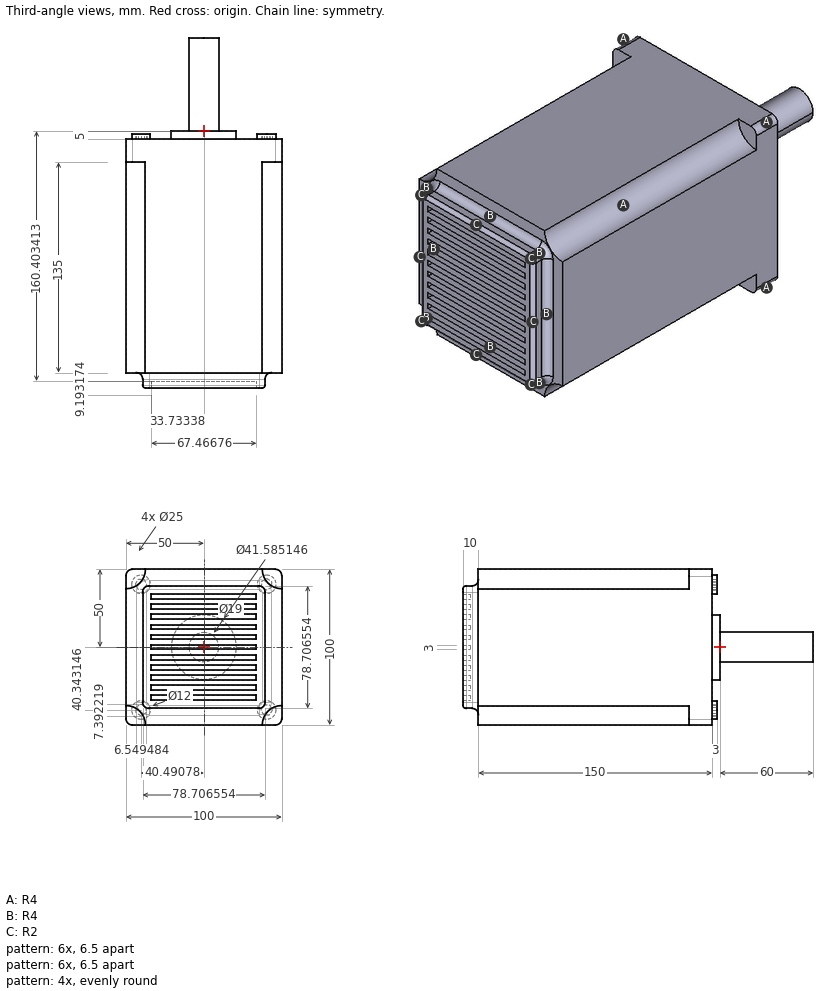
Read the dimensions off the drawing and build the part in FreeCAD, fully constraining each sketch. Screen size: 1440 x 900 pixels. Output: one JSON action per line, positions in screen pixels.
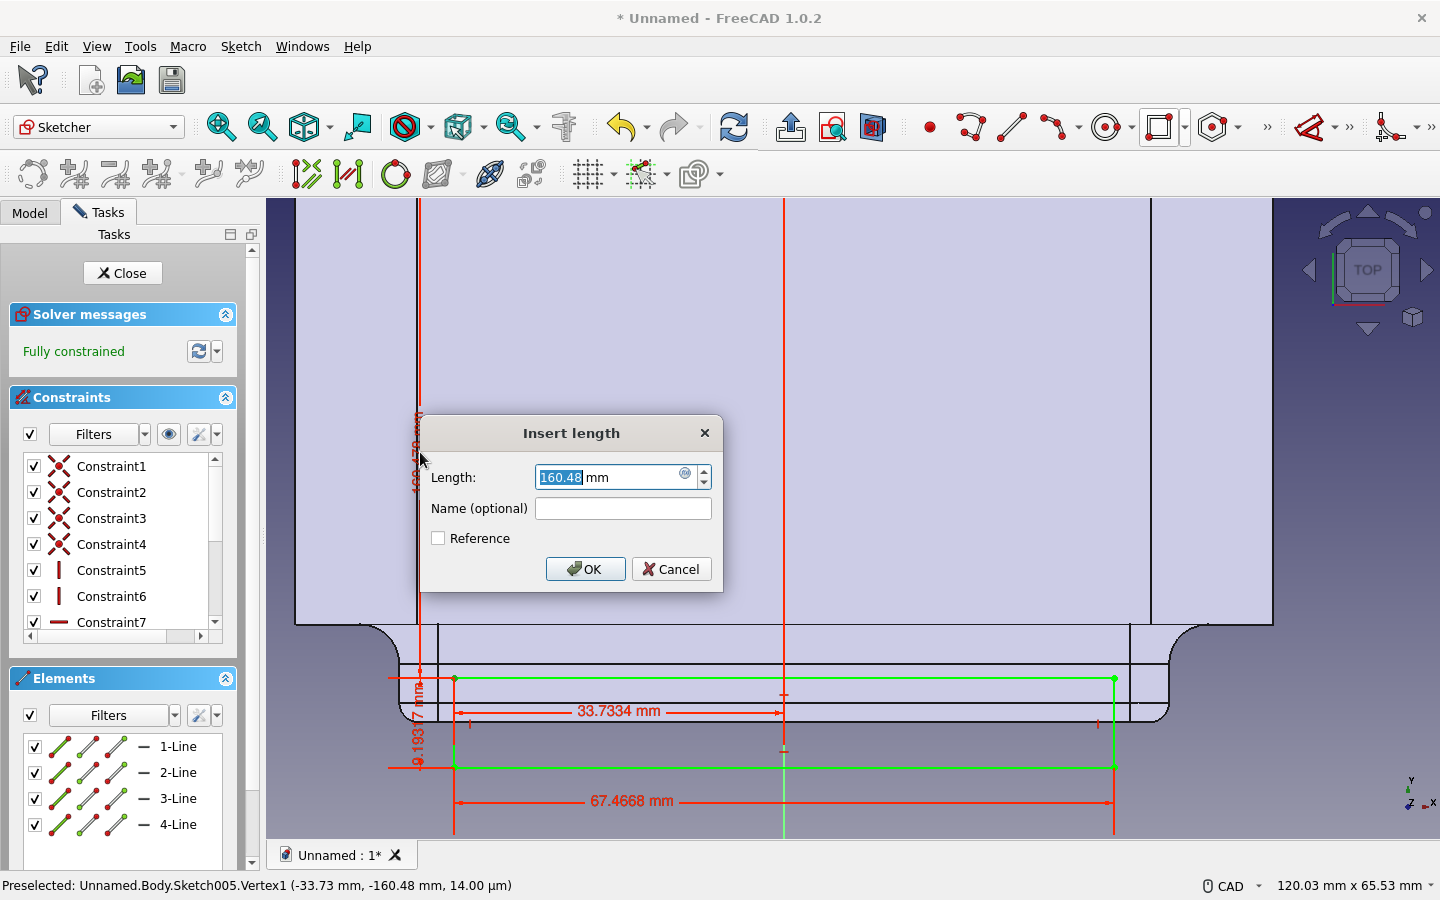
{"action": "type", "text": "160.403413"}
{"action": "key", "text": "Return"}
{"action": "key", "text": "Escape"}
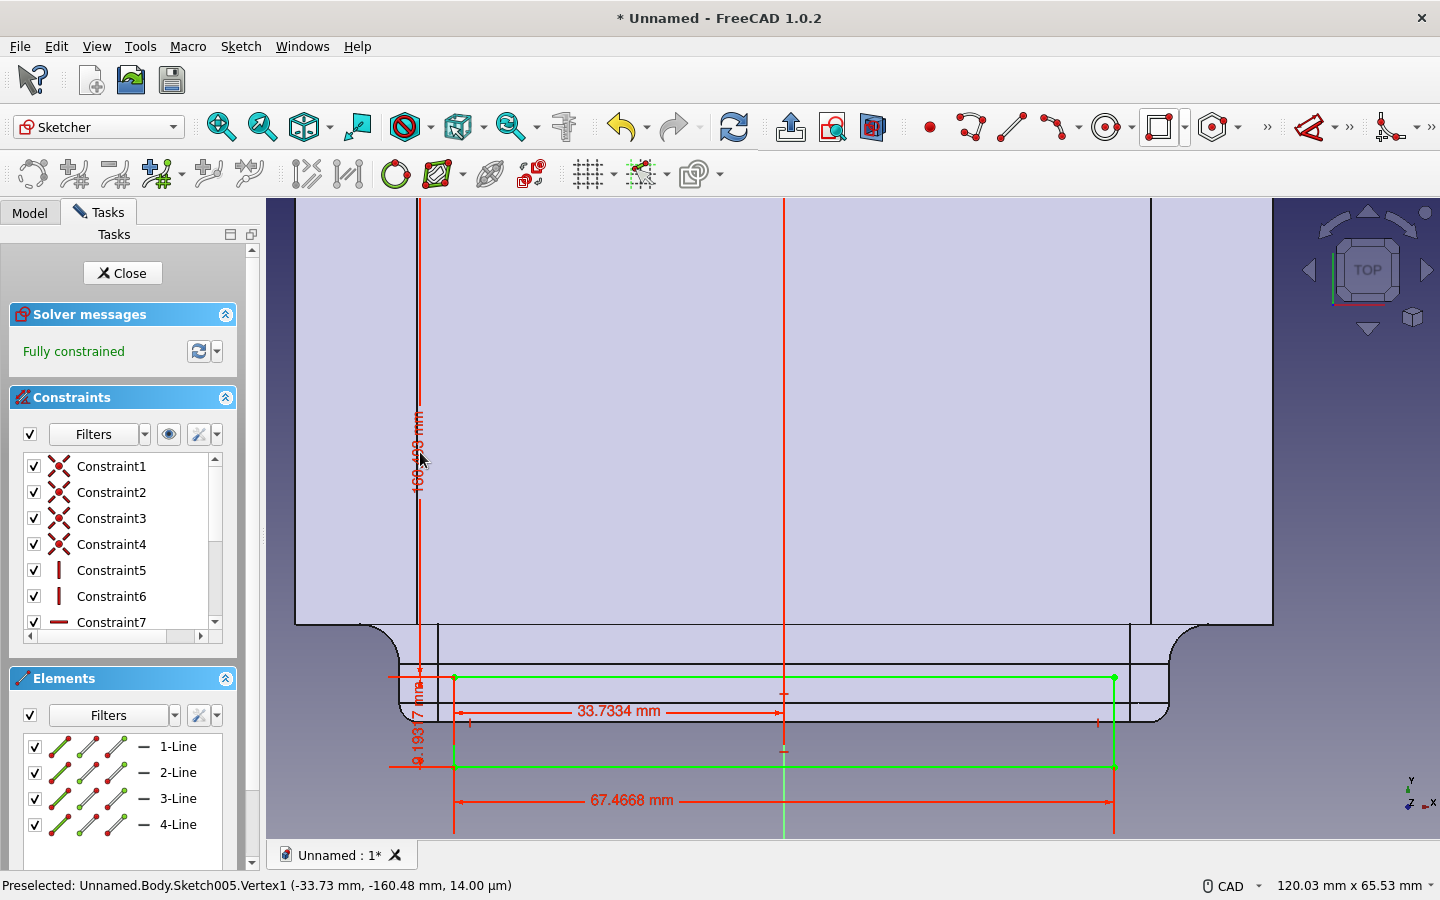
{"action": "left_click", "coordinate": [123, 273]}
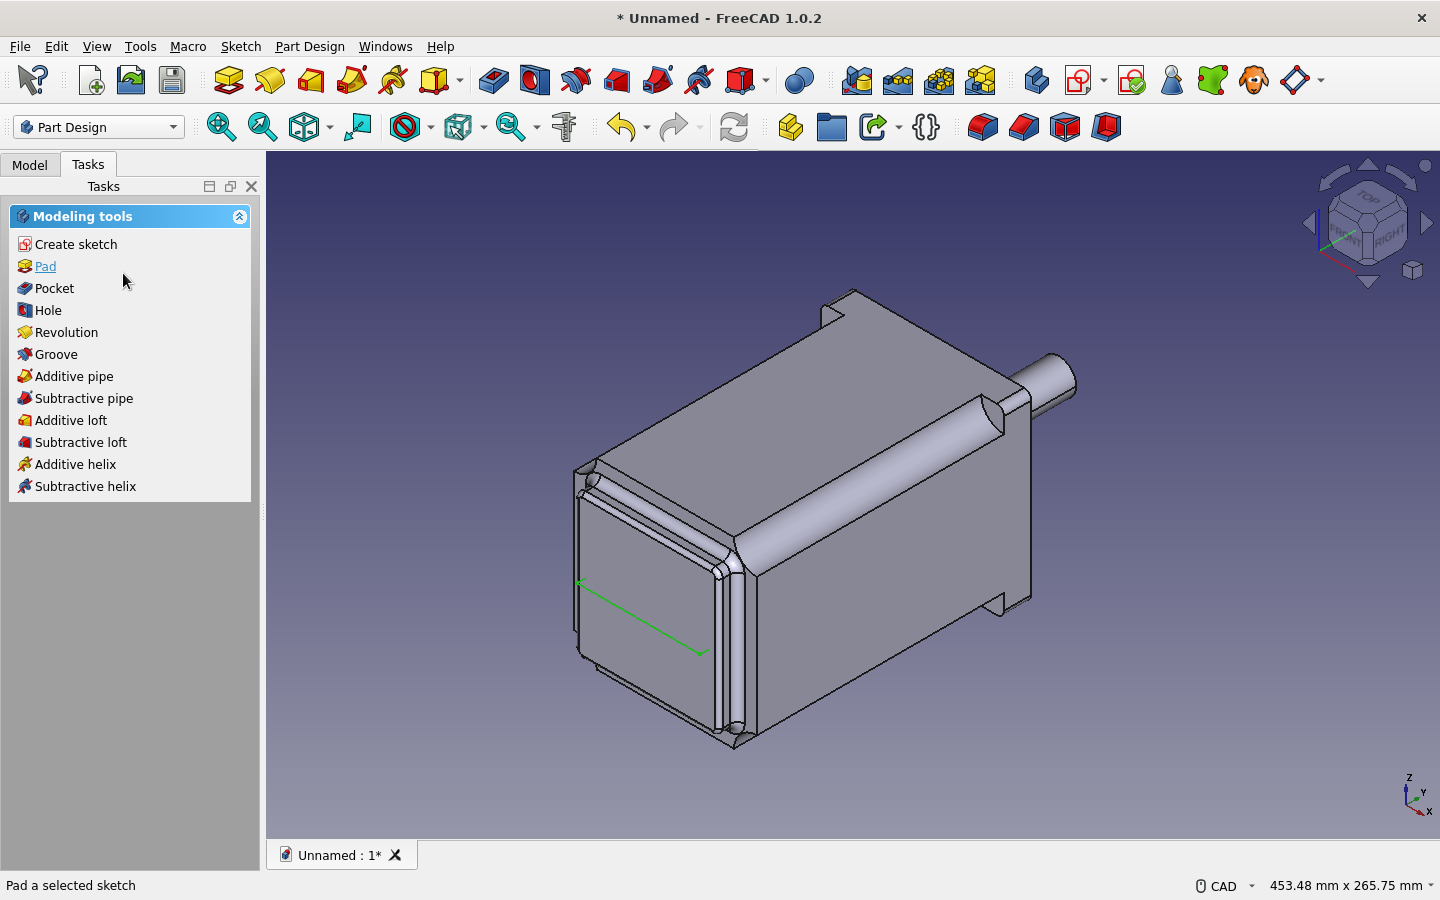
{"action": "left_click", "coordinate": [494, 80]}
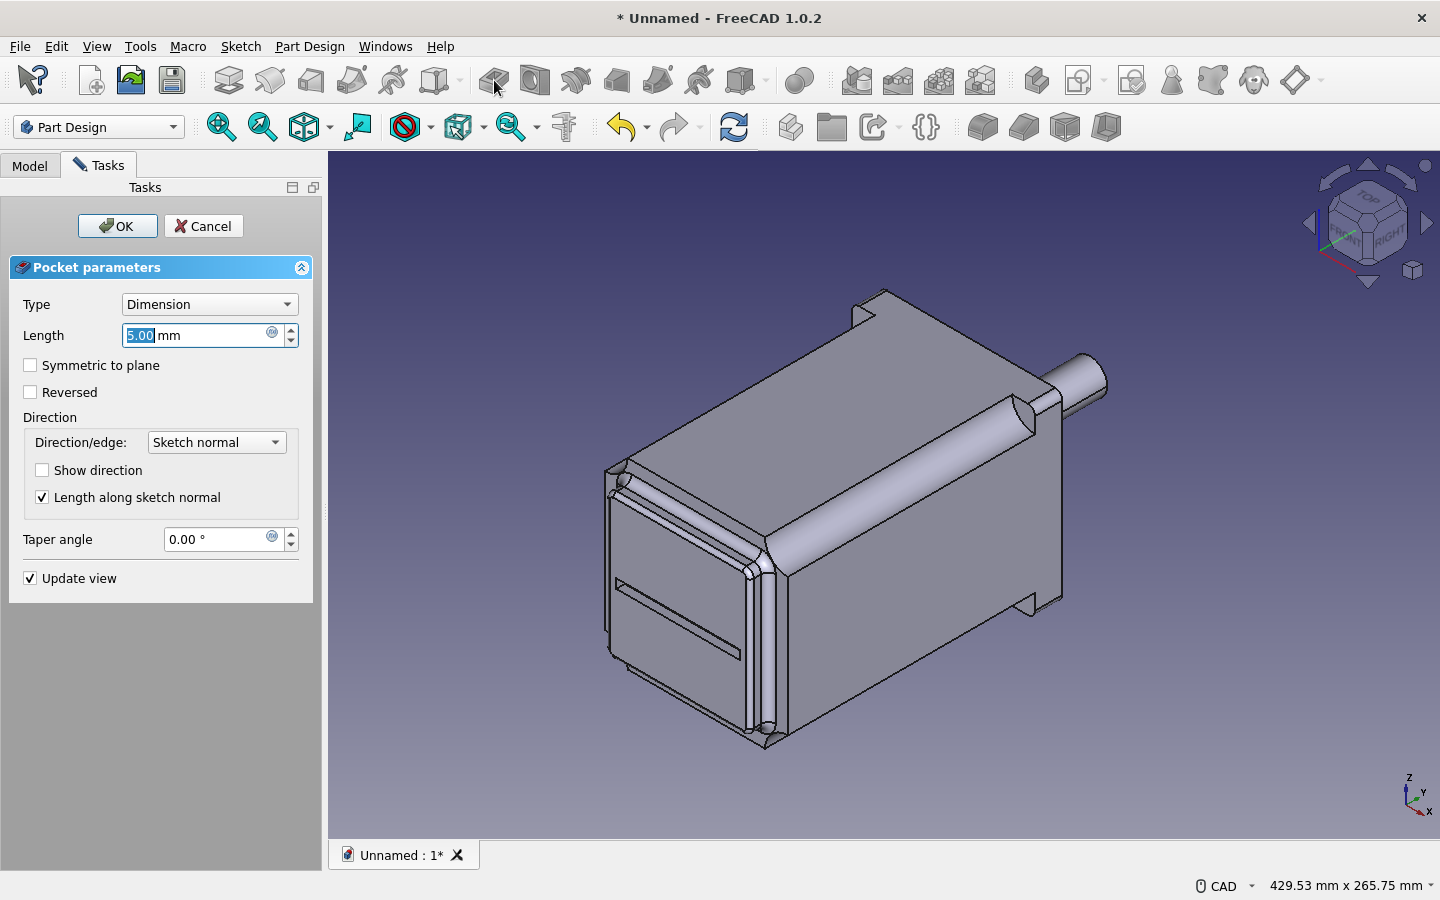
{"action": "type", "text": "3"}
{"action": "key", "text": "Tab"}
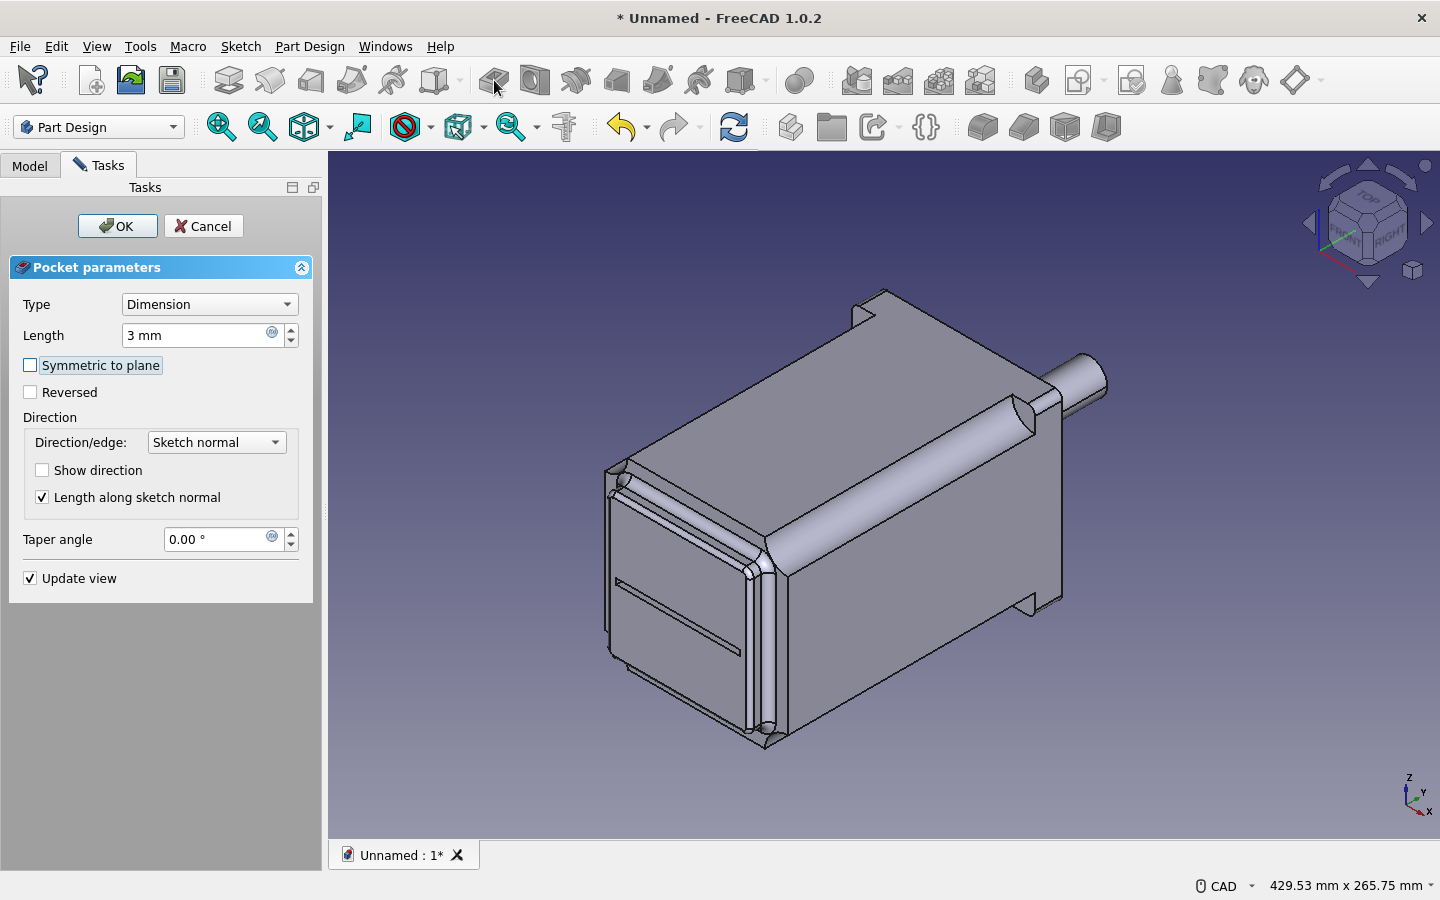
{"action": "left_click", "coordinate": [31, 365]}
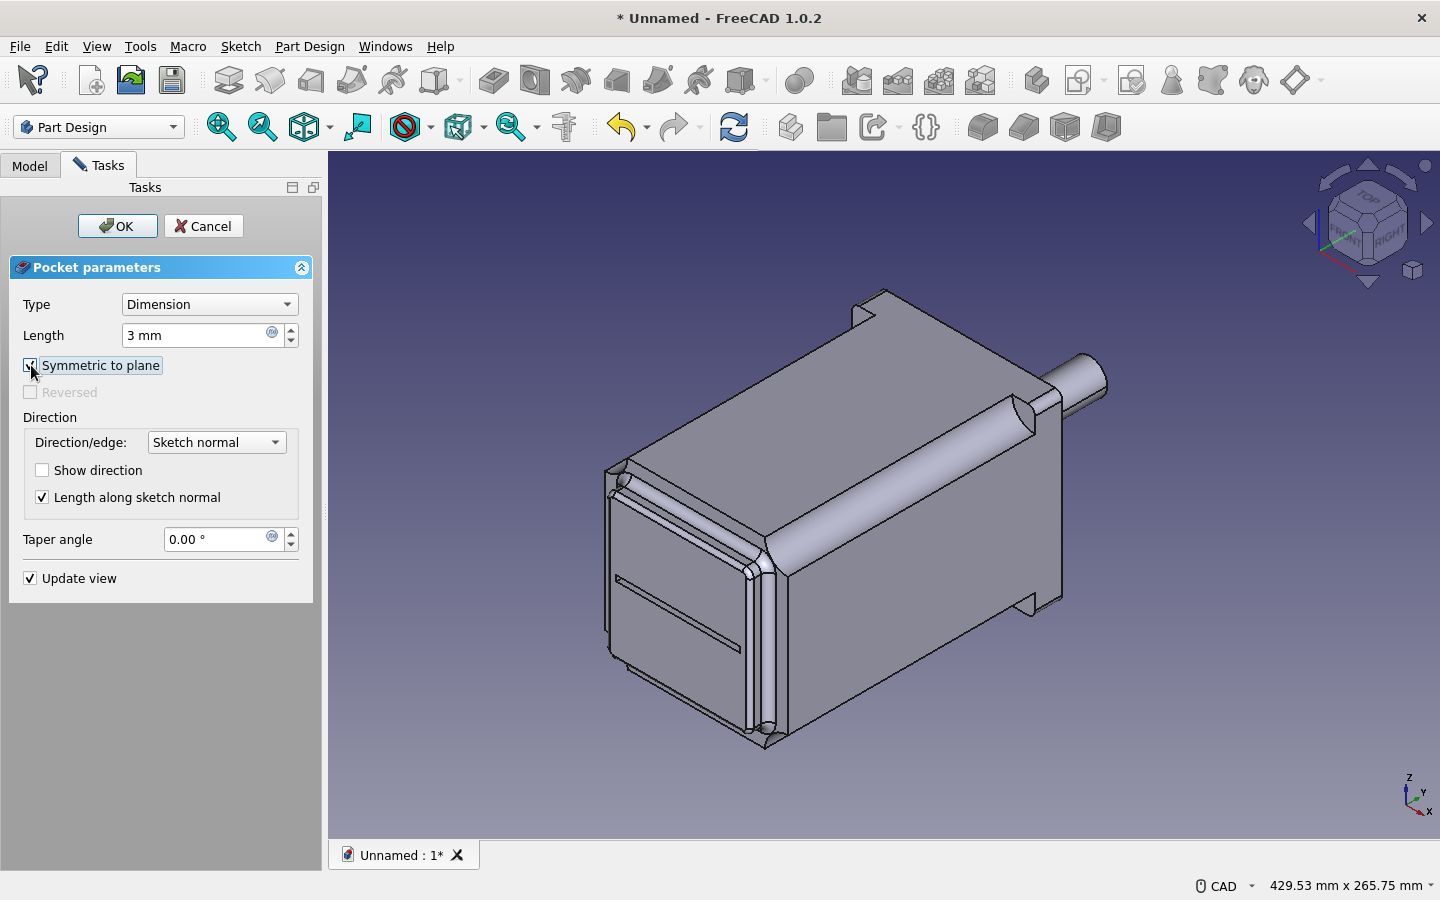
{"action": "left_click", "coordinate": [118, 226]}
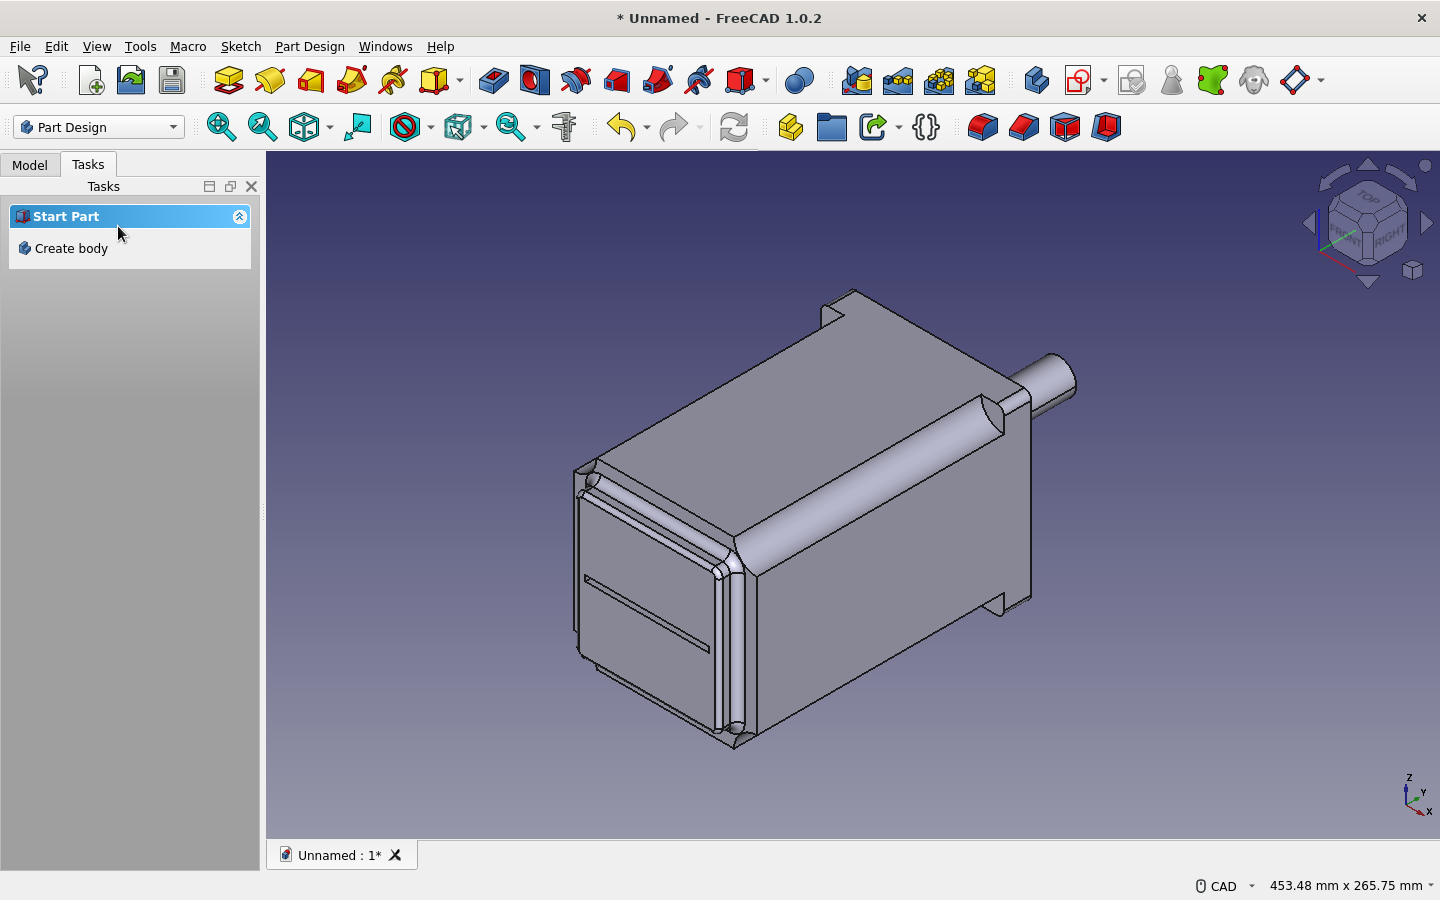
{"action": "left_click", "coordinate": [30, 164]}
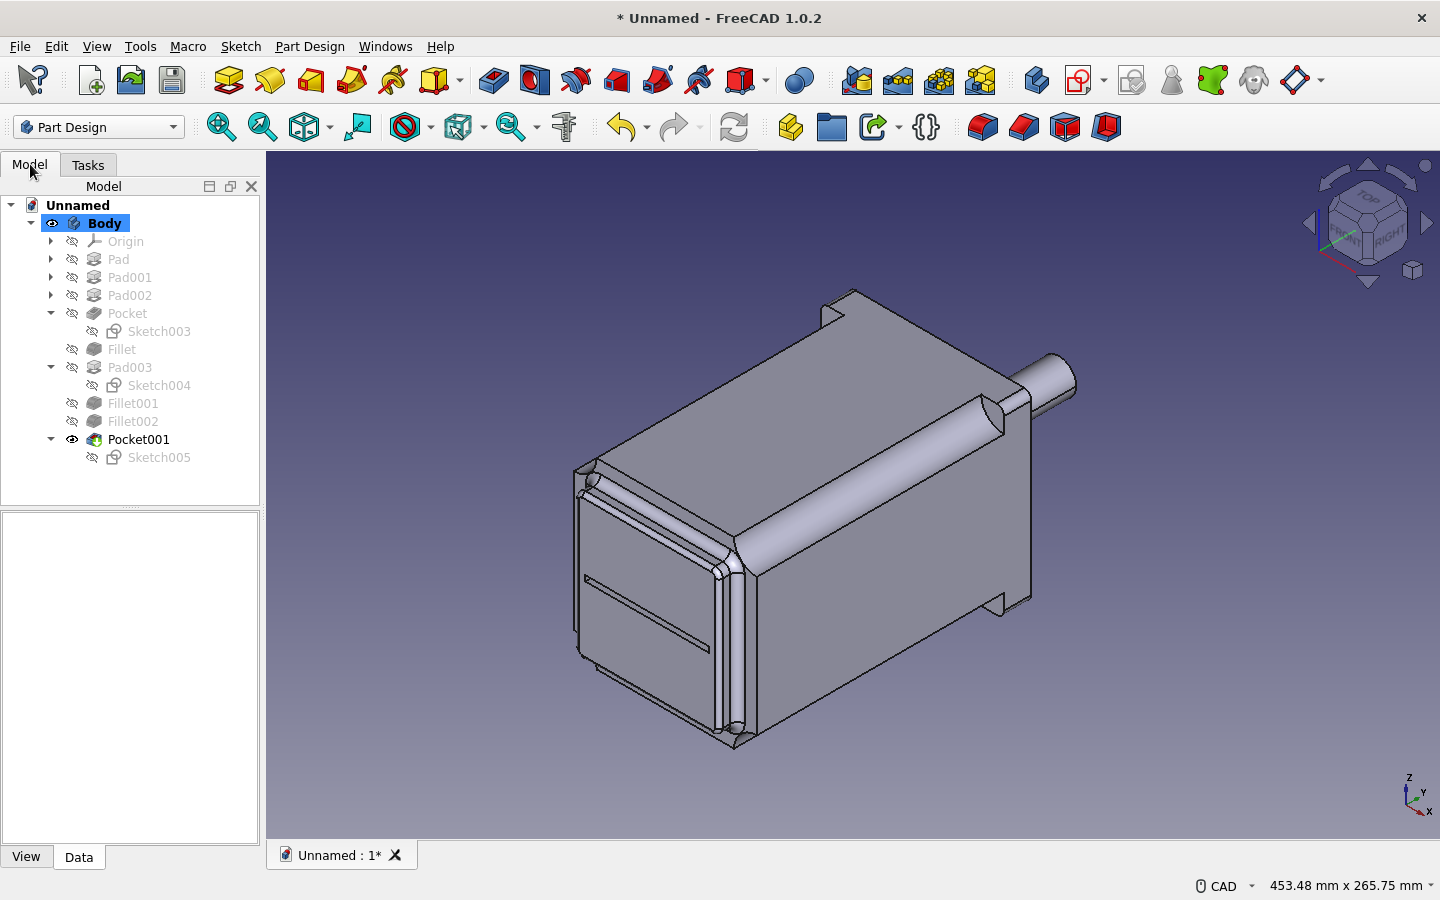
{"action": "left_click", "coordinate": [117, 439]}